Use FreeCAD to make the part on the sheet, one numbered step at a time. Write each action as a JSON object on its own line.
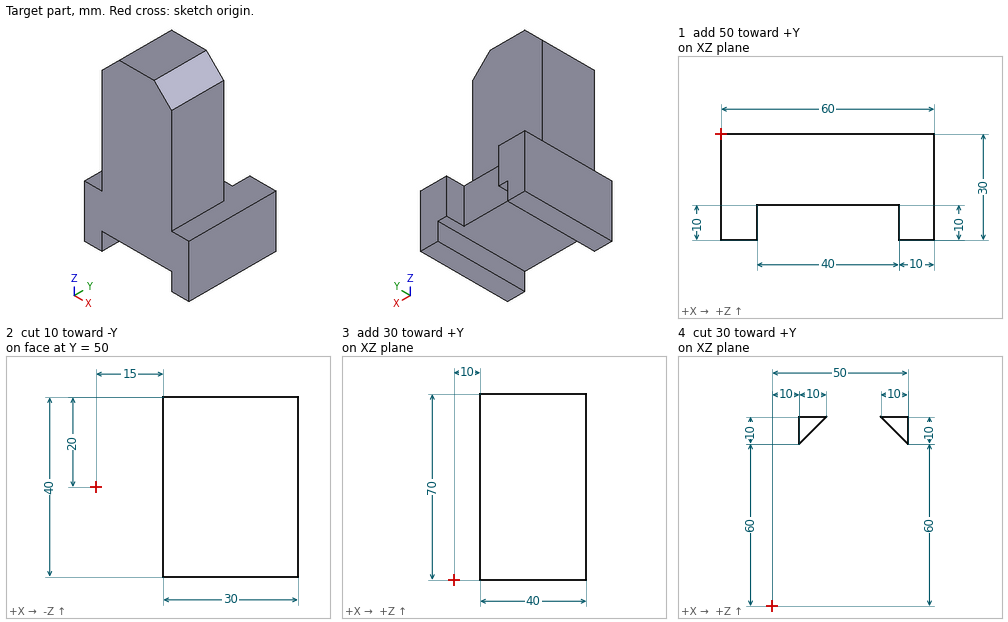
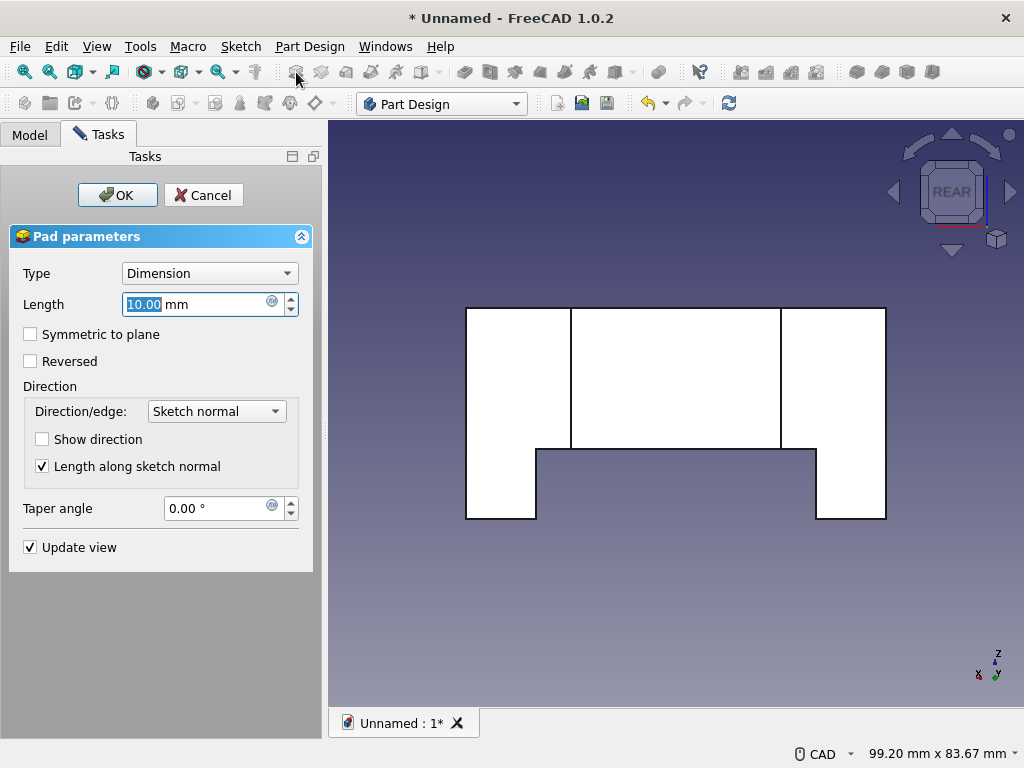
{"action": "type", "text": "30"}
{"action": "key", "text": "Tab"}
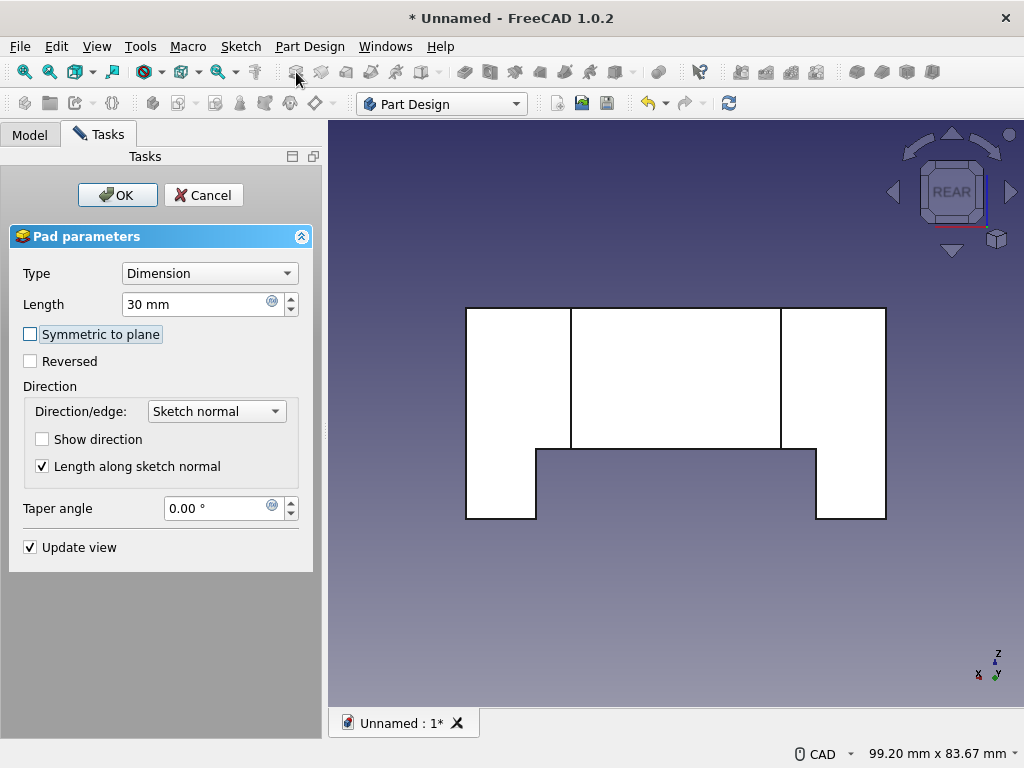
{"action": "left_click", "coordinate": [31, 361]}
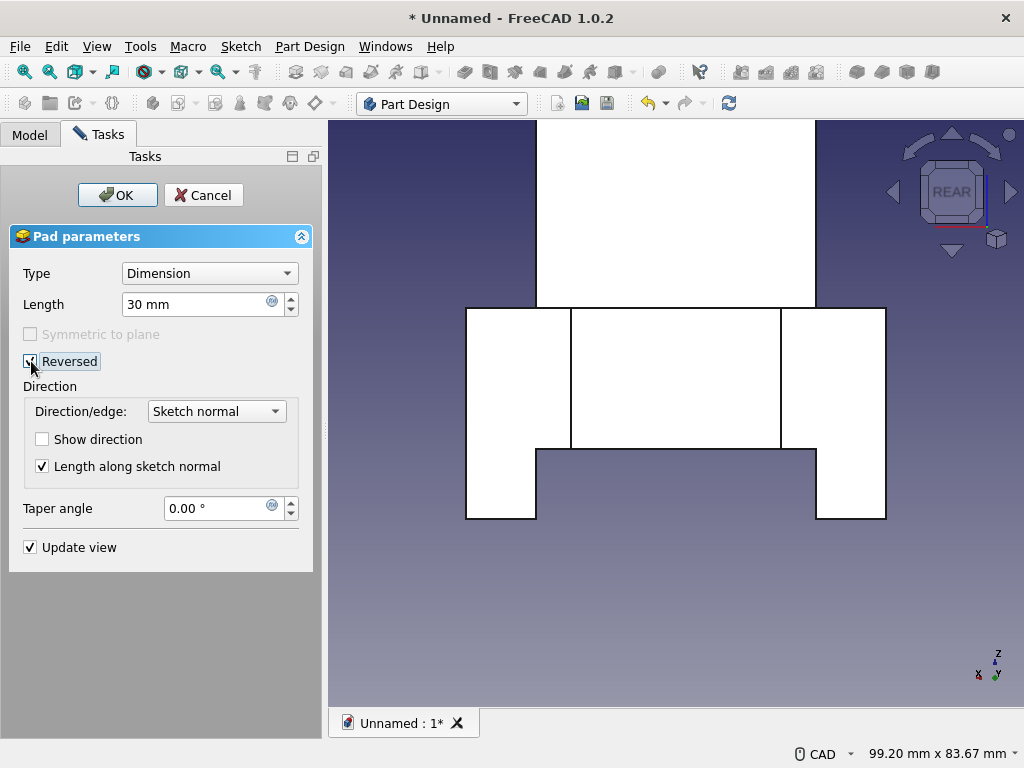
{"action": "left_click", "coordinate": [118, 195]}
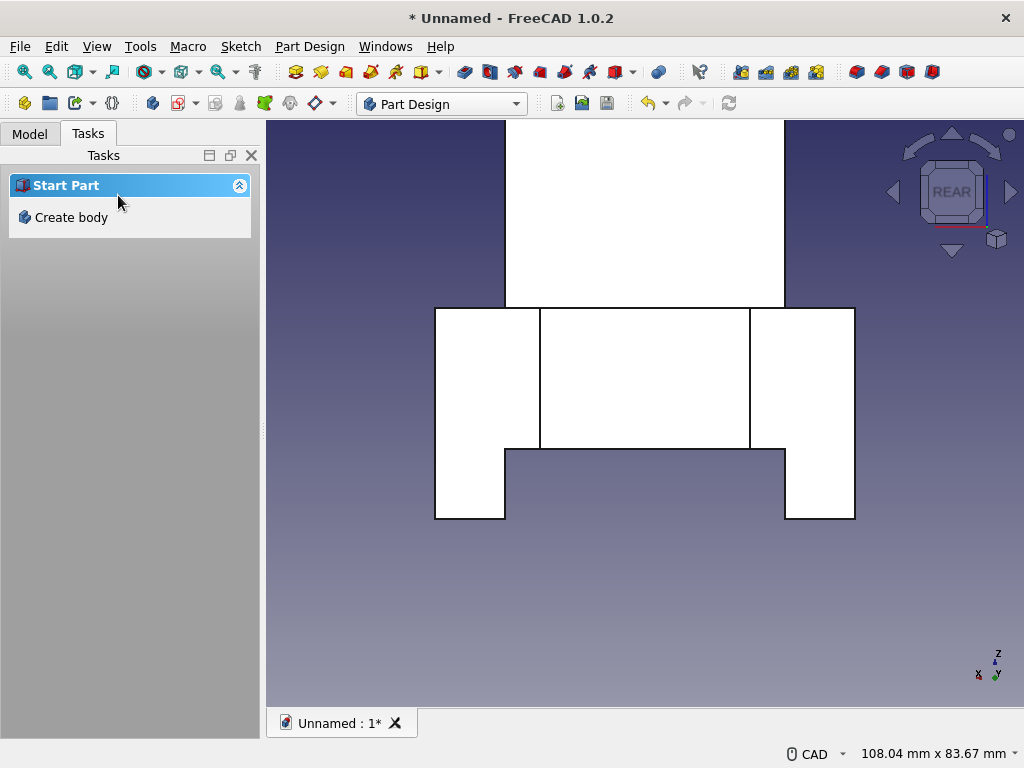
{"action": "left_click", "coordinate": [25, 72]}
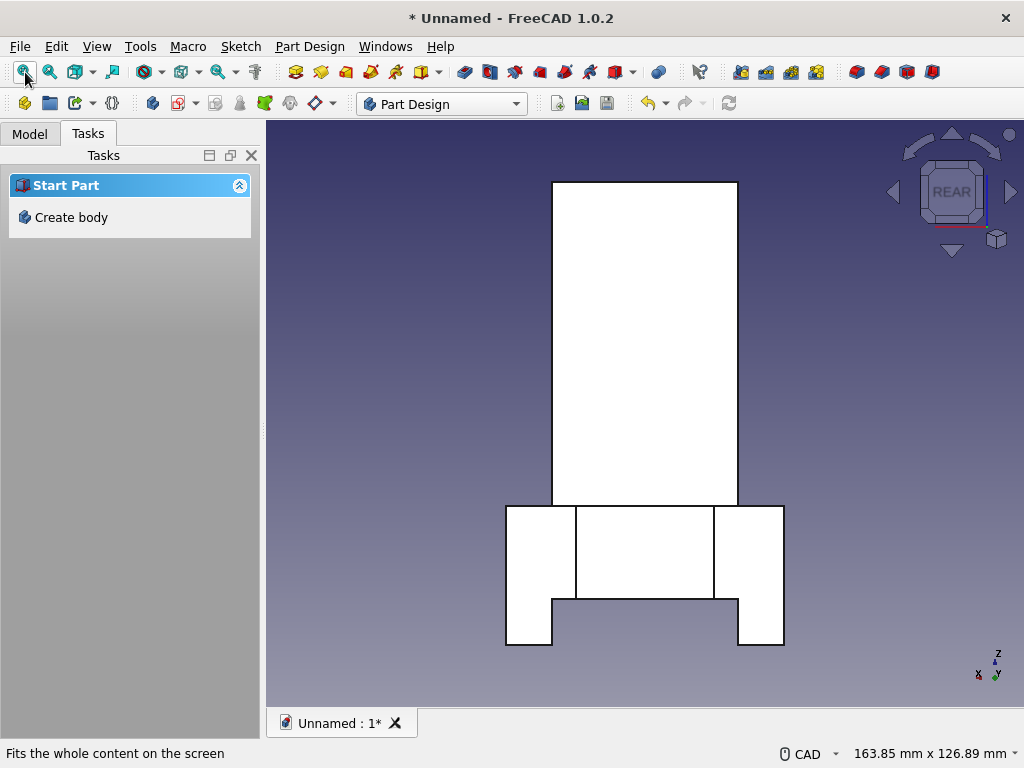
{"action": "left_click", "coordinate": [178, 104]}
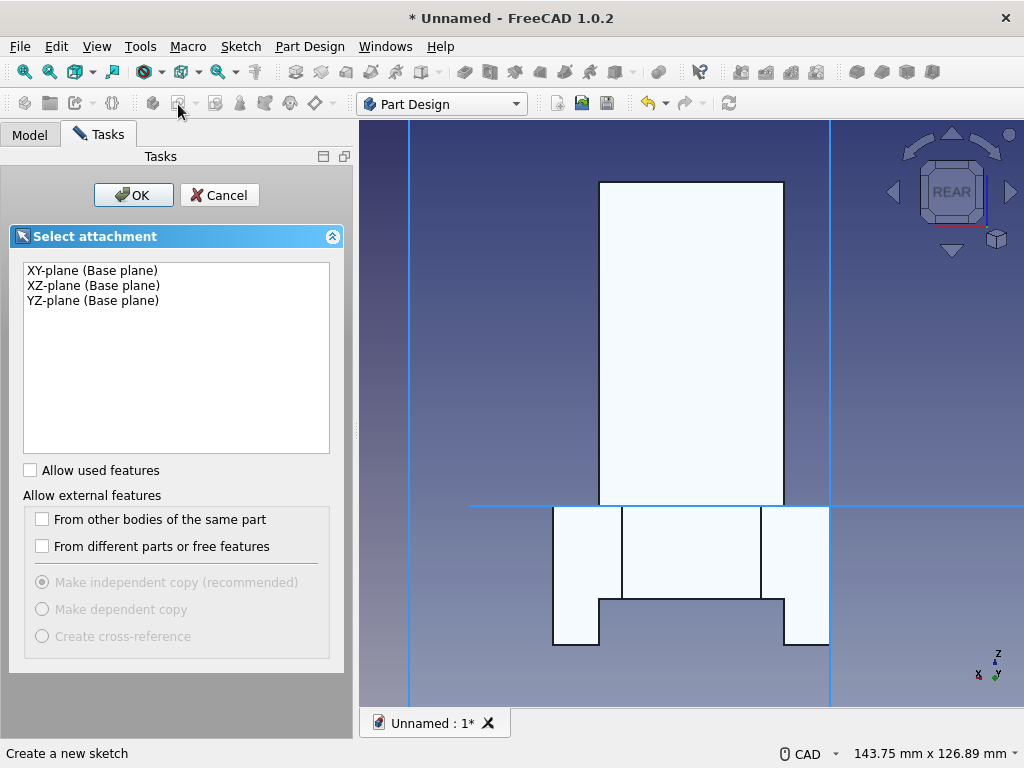
{"action": "left_click", "coordinate": [84, 286]}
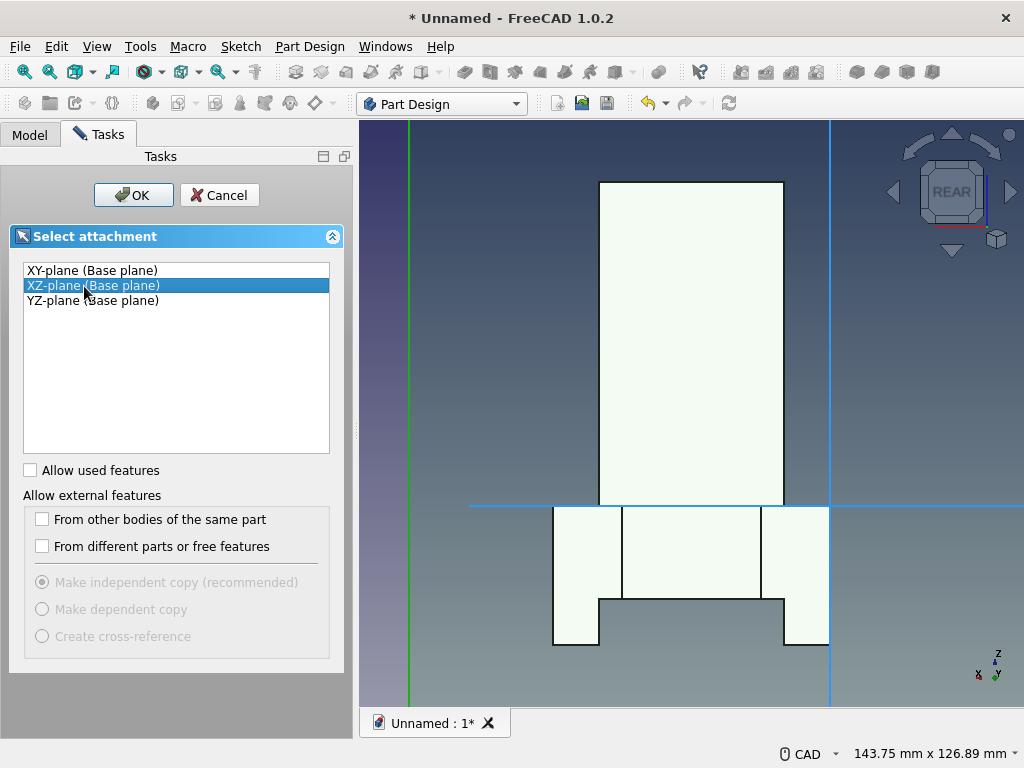
{"action": "left_click", "coordinate": [134, 195]}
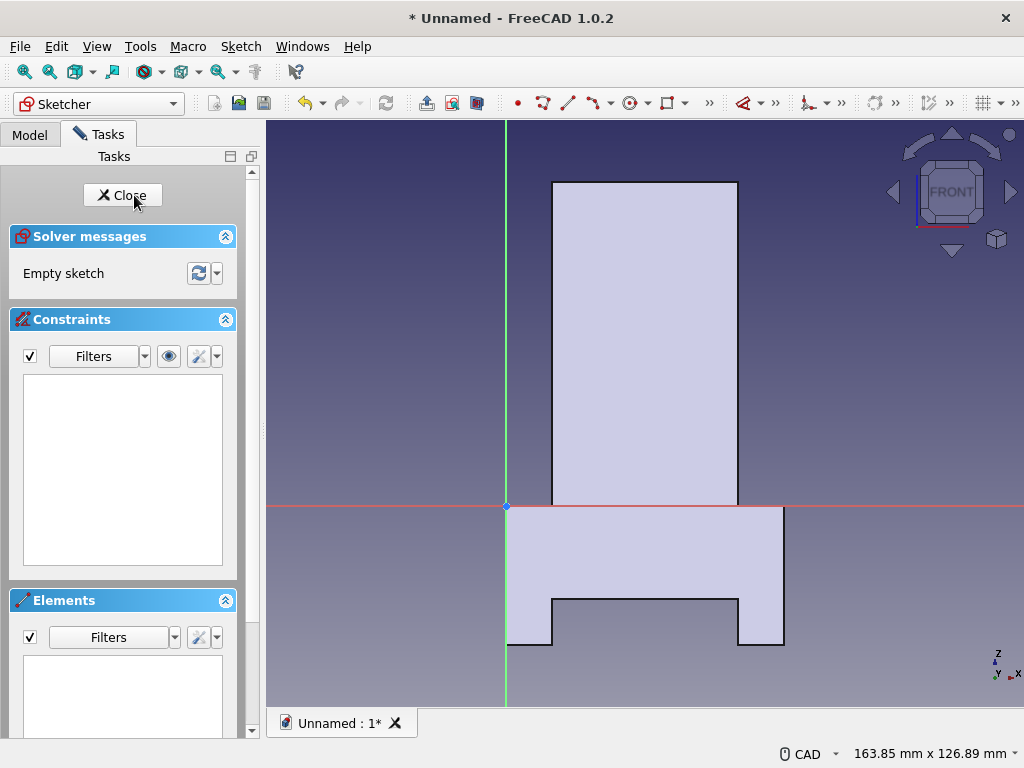
{"action": "key", "text": "g m"}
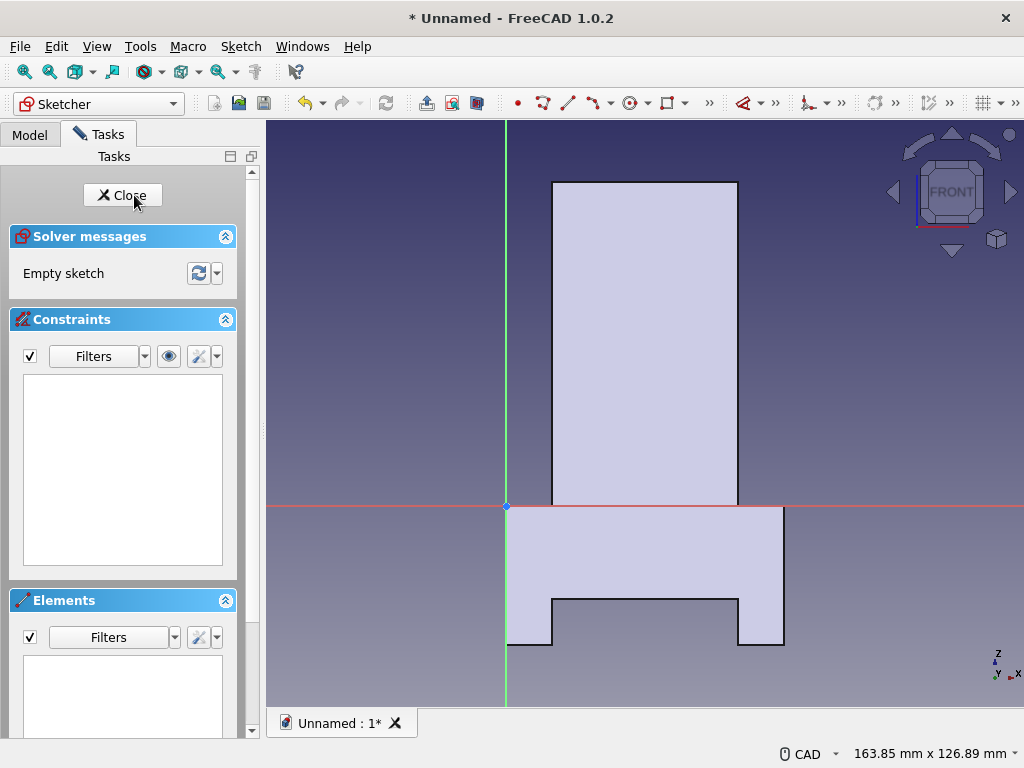
{"action": "left_click", "coordinate": [738, 228]}
{"action": "left_click", "coordinate": [738, 182]}
{"action": "left_click", "coordinate": [691, 182]}
{"action": "left_click", "coordinate": [738, 229]}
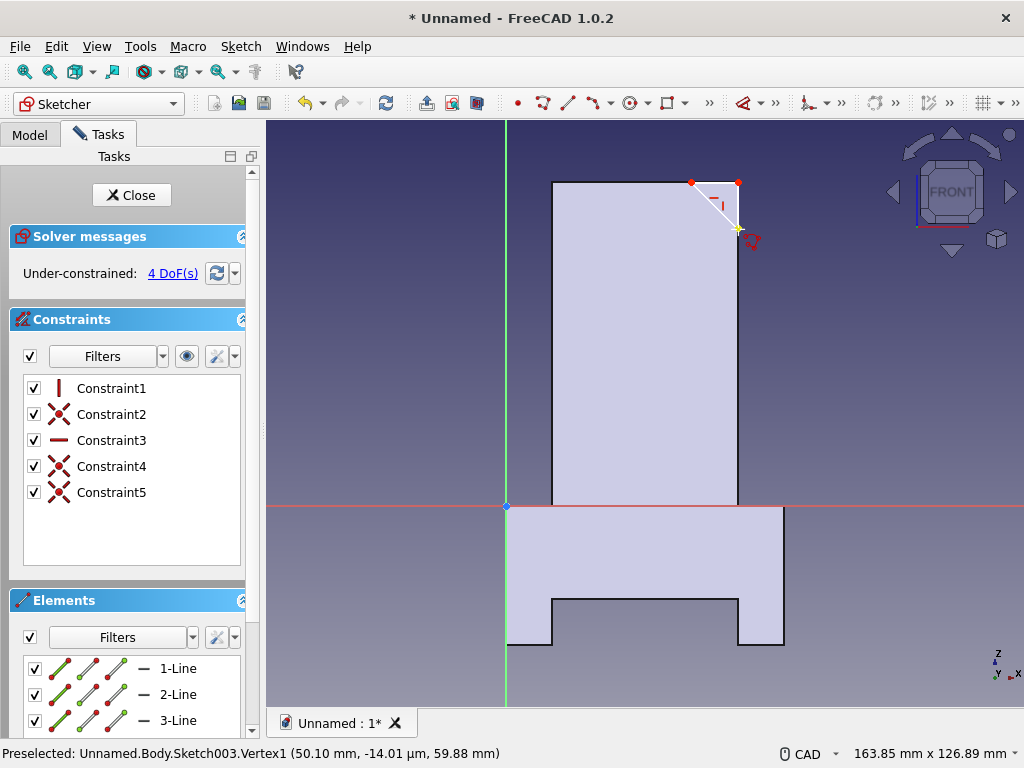
{"action": "left_click", "coordinate": [552, 228]}
{"action": "left_click", "coordinate": [599, 182]}
{"action": "left_click", "coordinate": [552, 182]}
{"action": "left_click", "coordinate": [552, 229]}
{"action": "key", "text": "Escape"}
{"action": "key", "text": "Escape"}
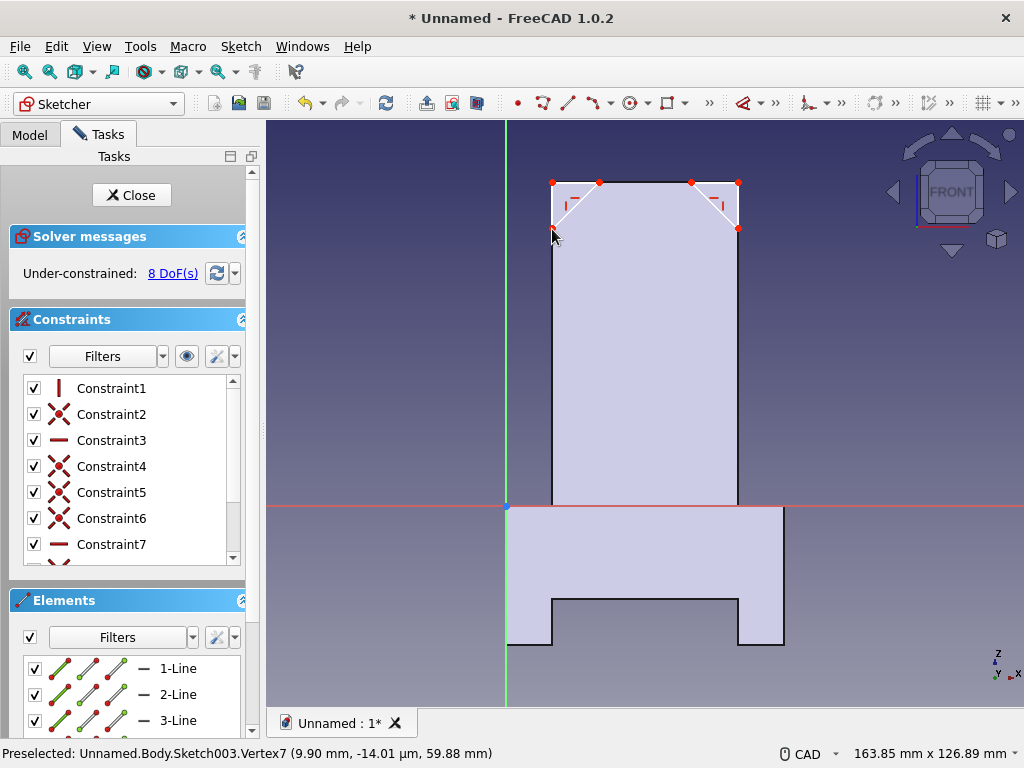
{"action": "left_click", "coordinate": [742, 104]}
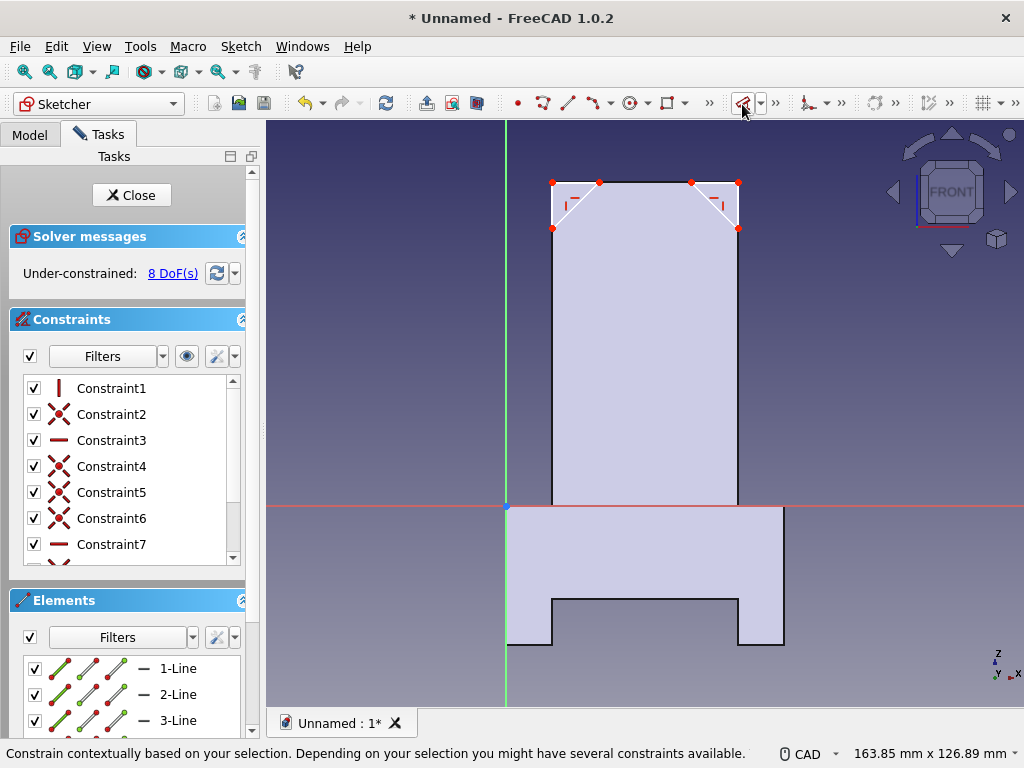
{"action": "scroll", "coordinate": [738, 215], "scroll_direction": "up", "scroll_amount": 2}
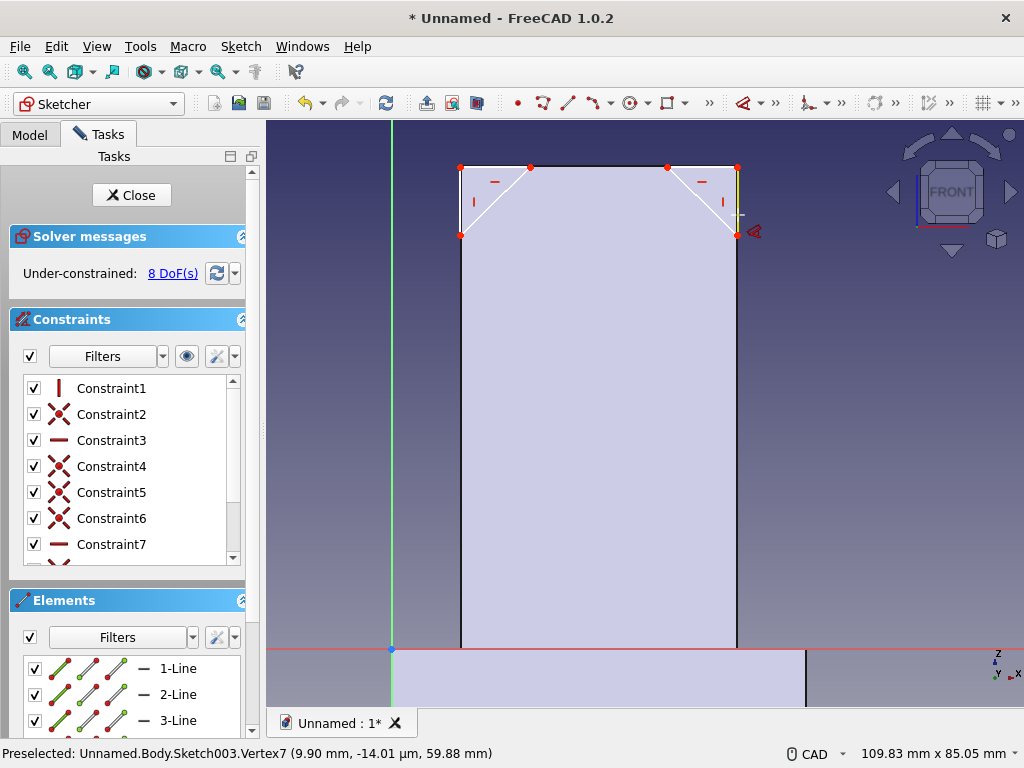
{"action": "left_click", "coordinate": [738, 215]}
{"action": "left_click", "coordinate": [772, 201]}